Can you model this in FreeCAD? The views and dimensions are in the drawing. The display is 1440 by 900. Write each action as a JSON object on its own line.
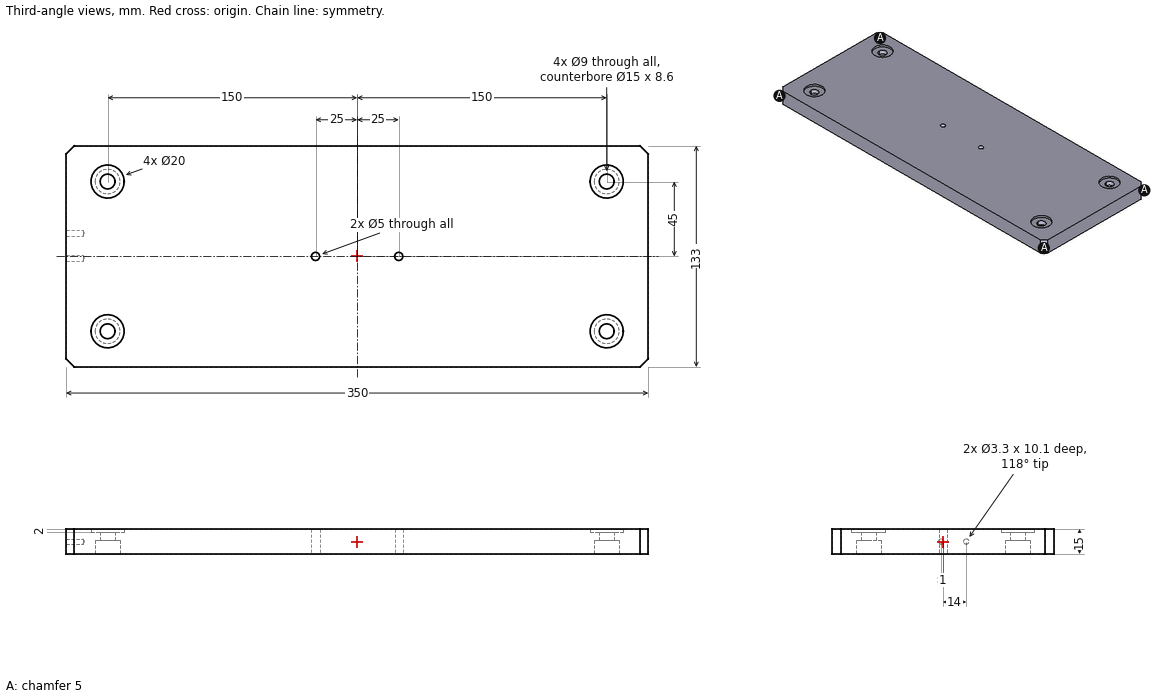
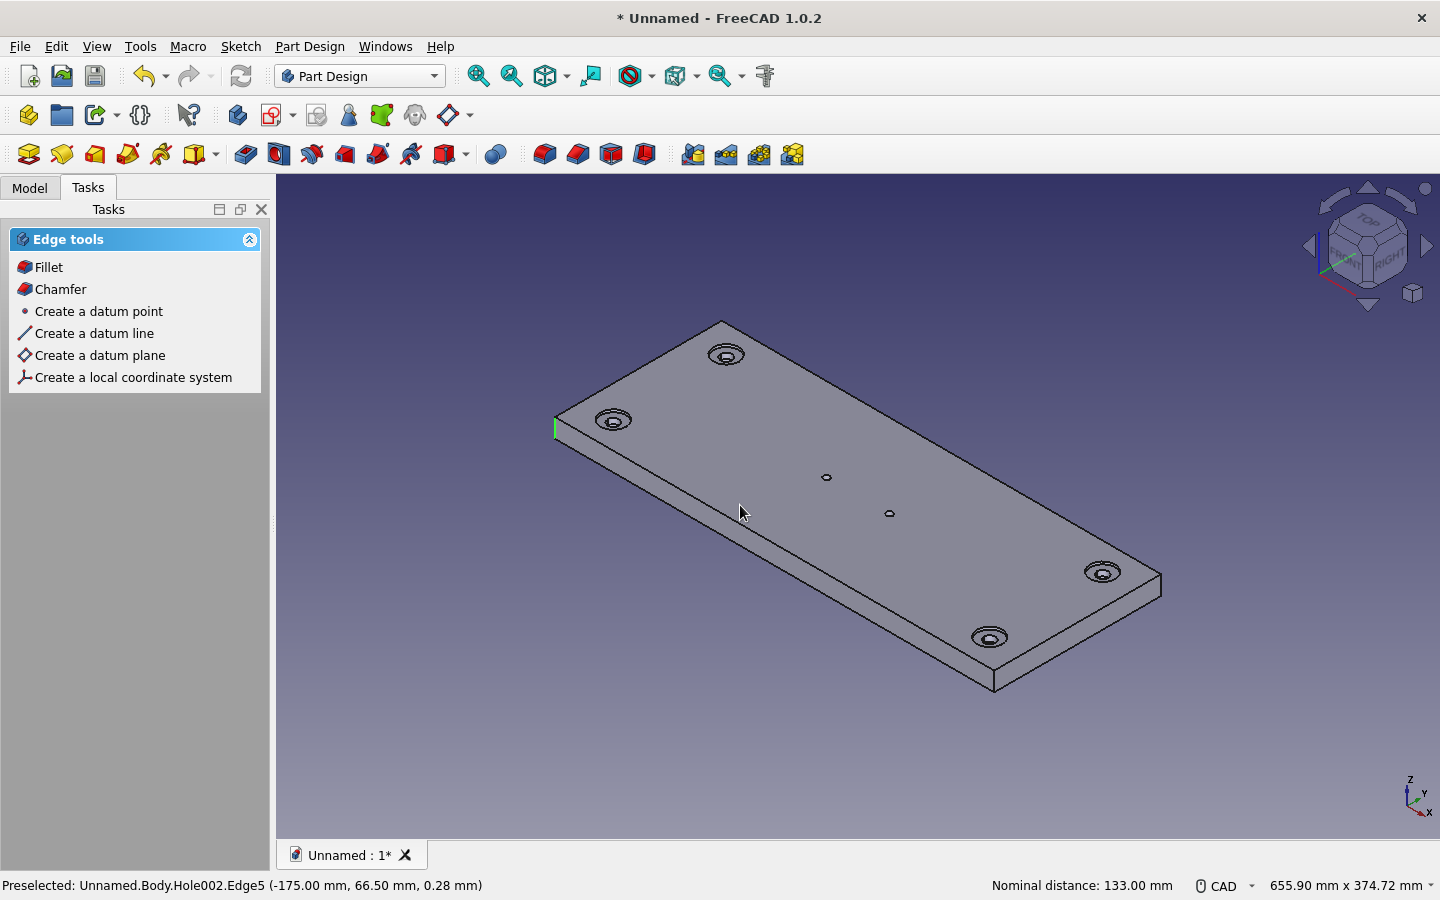
{"action": "left_click", "coordinate": [994, 680], "text": "ctrl"}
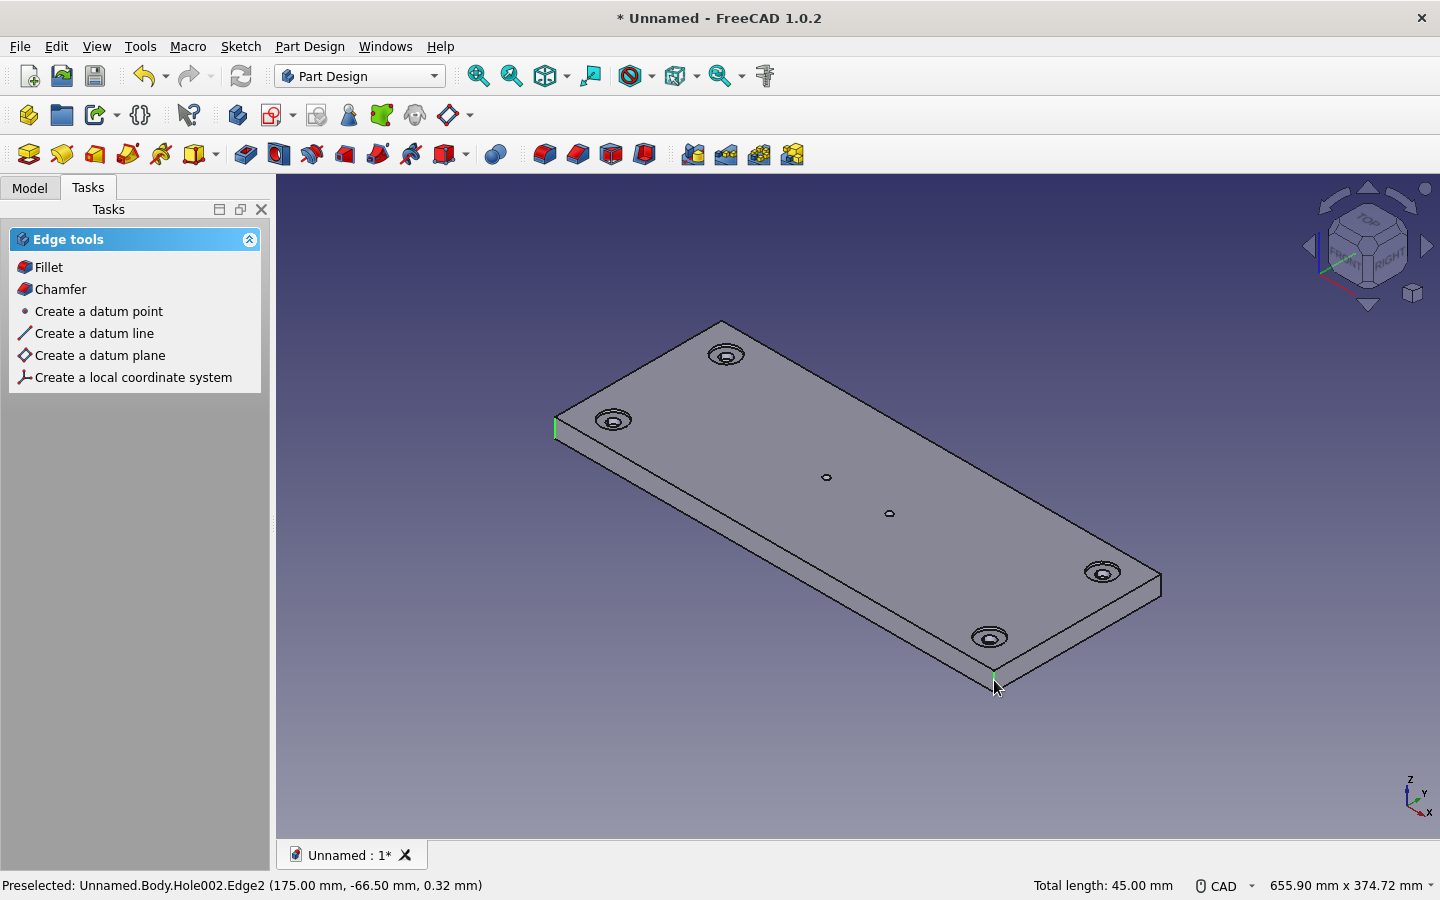
{"action": "key", "text": "2"}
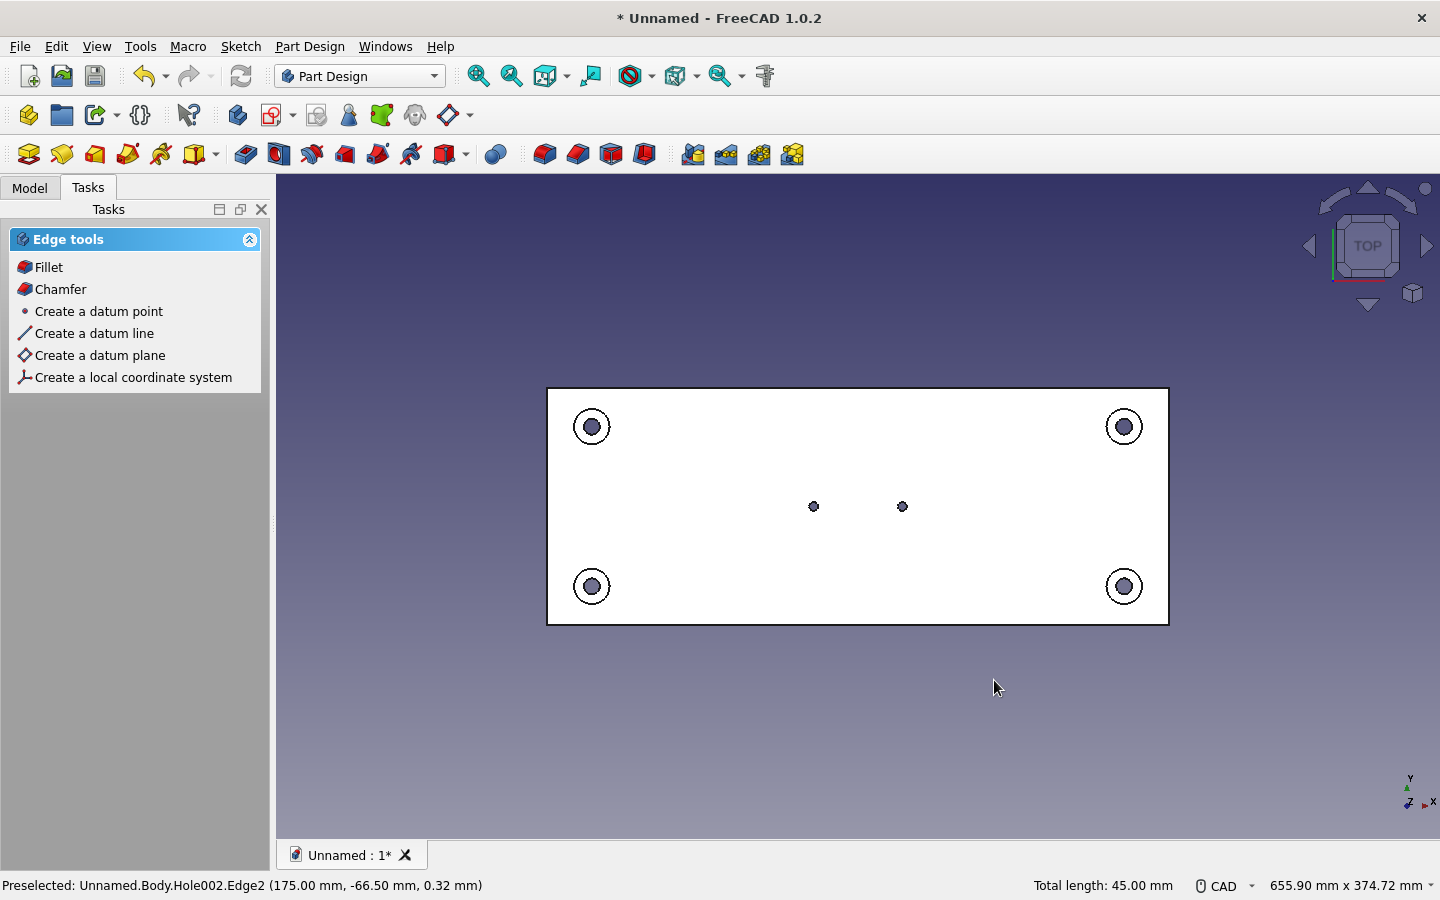
{"action": "key", "text": "1"}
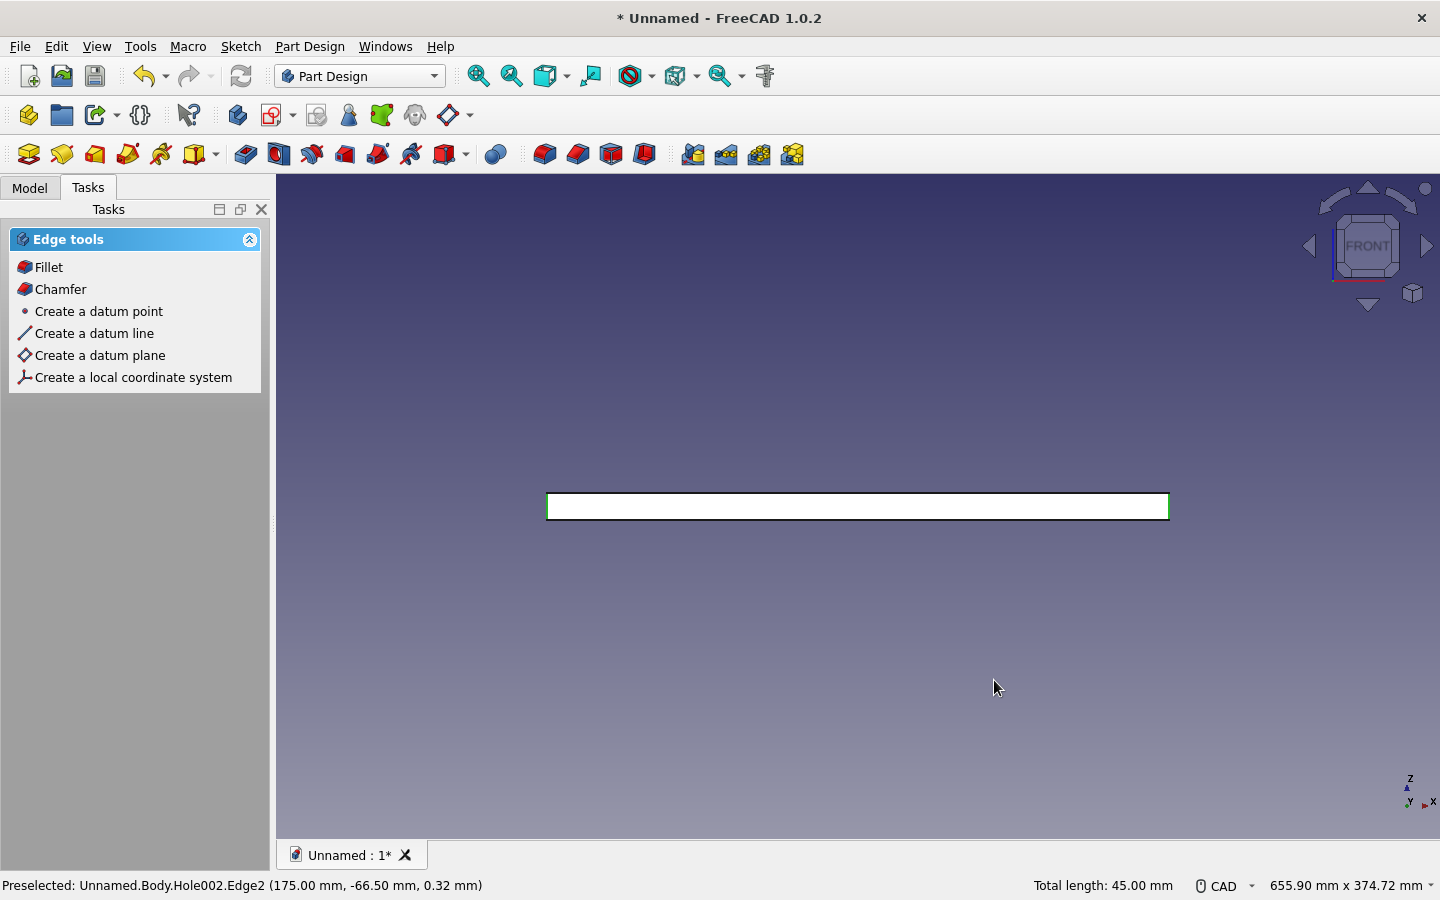
{"action": "key", "text": "3"}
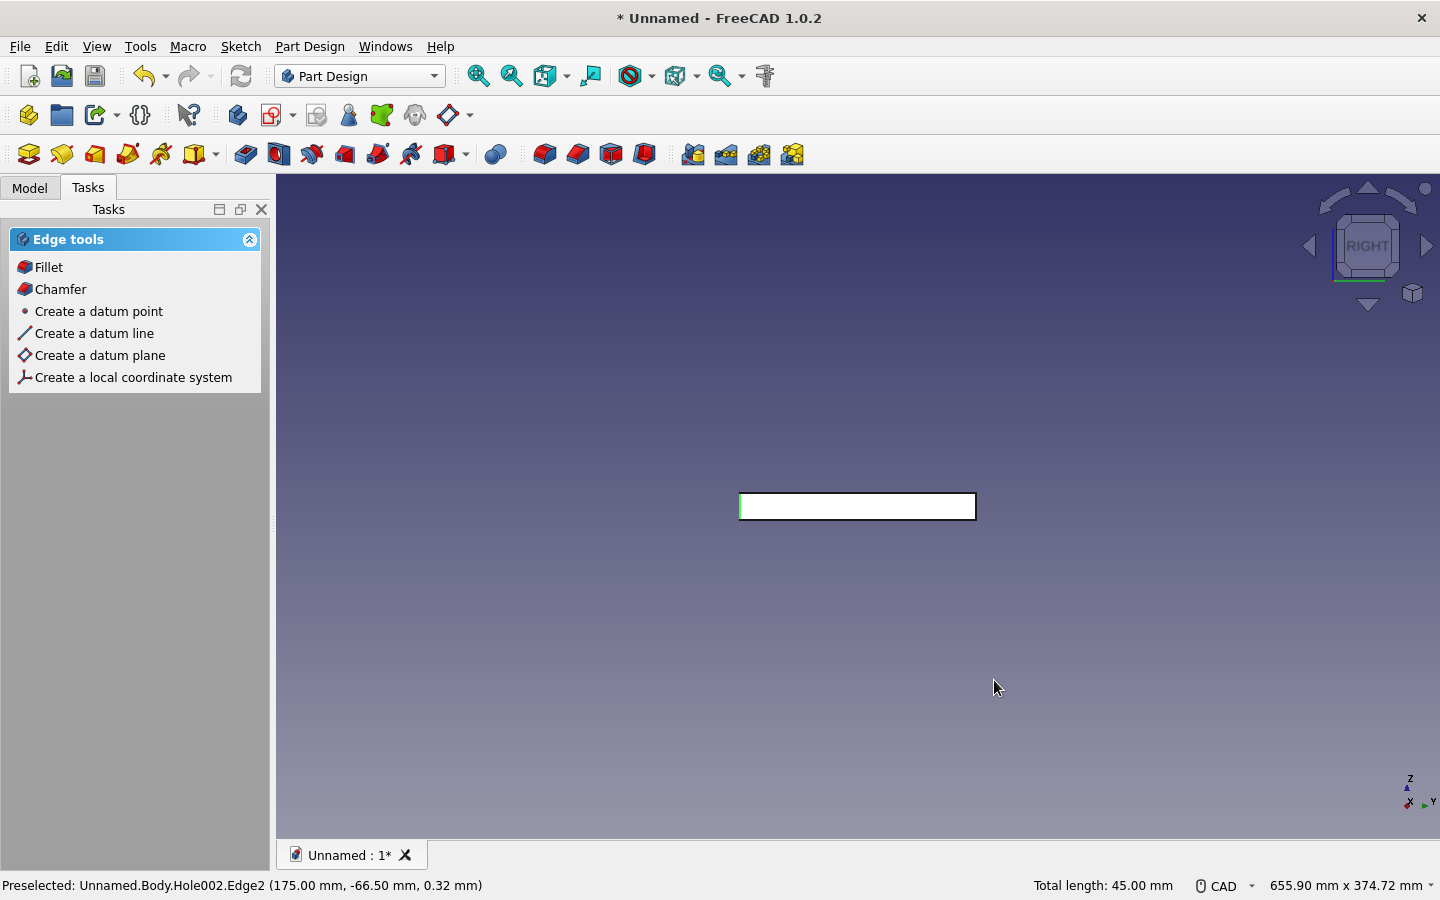
{"action": "key", "text": "v f"}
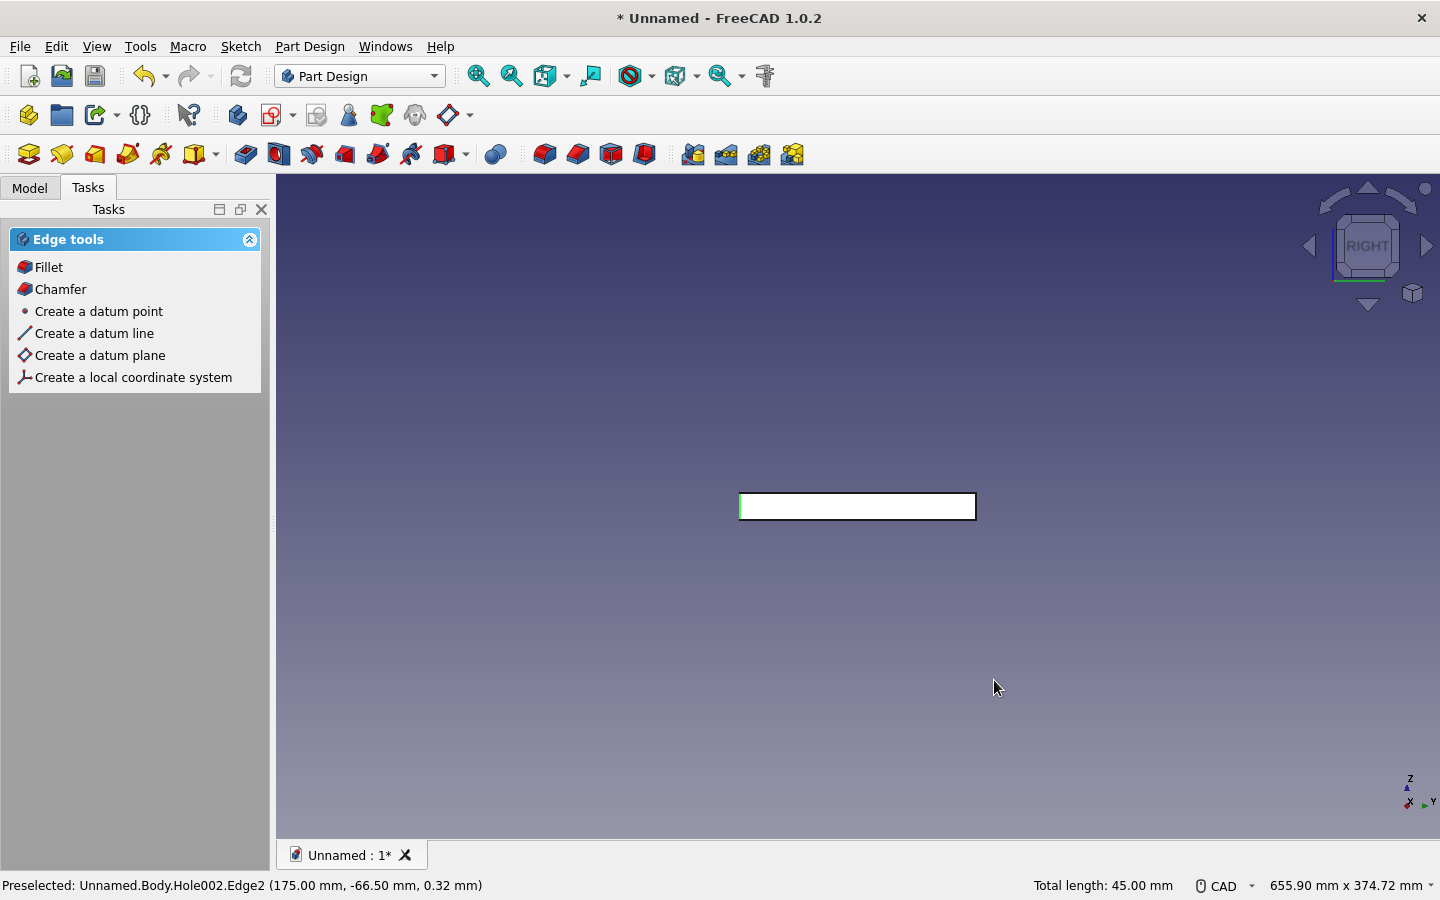
{"action": "left_click", "coordinate": [976, 505], "text": "ctrl"}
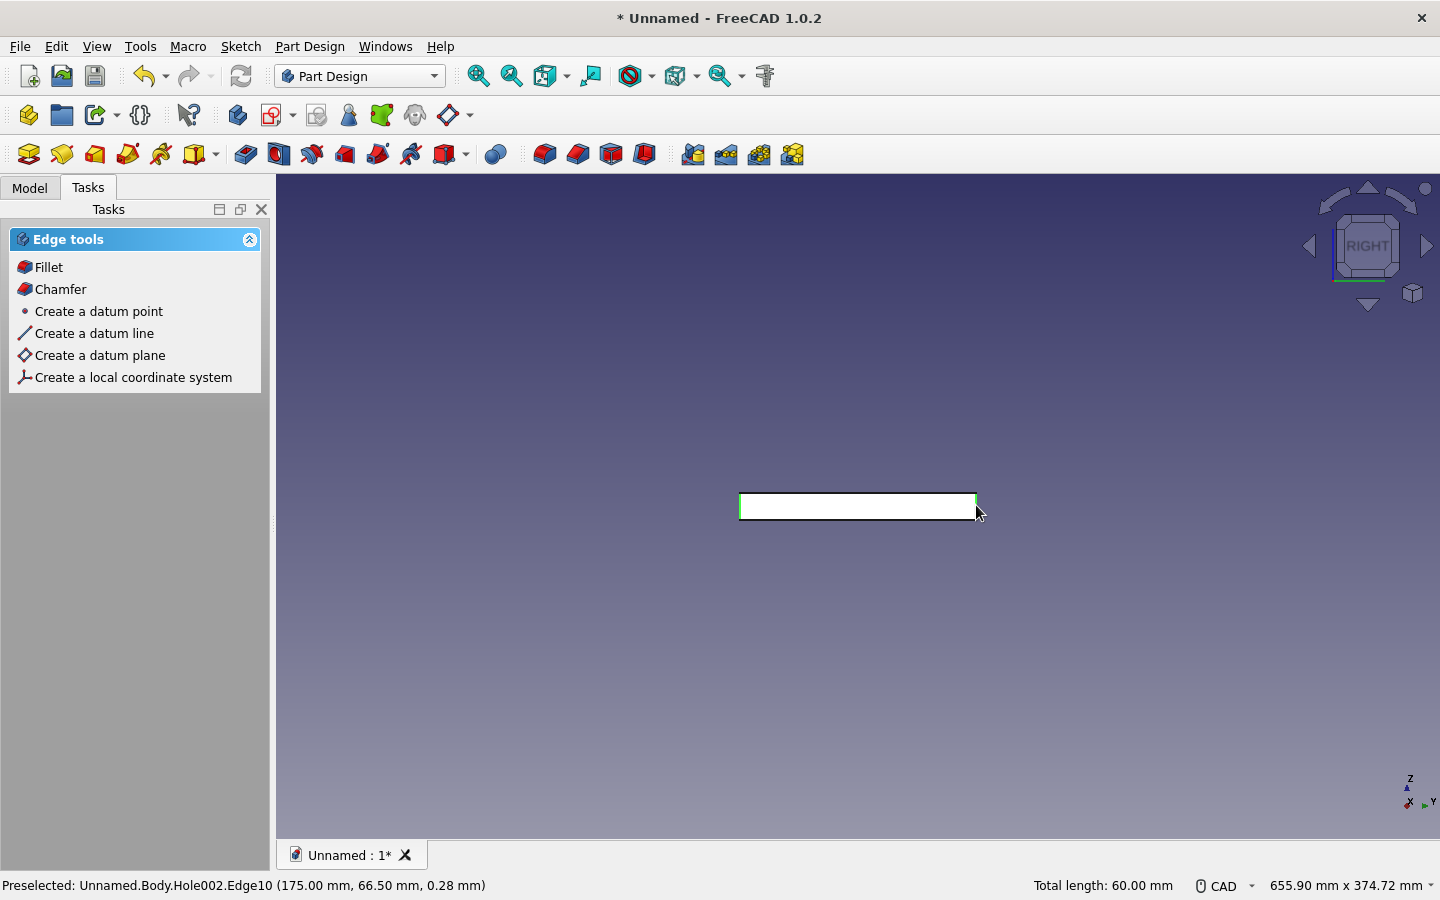
{"action": "left_click", "coordinate": [578, 154]}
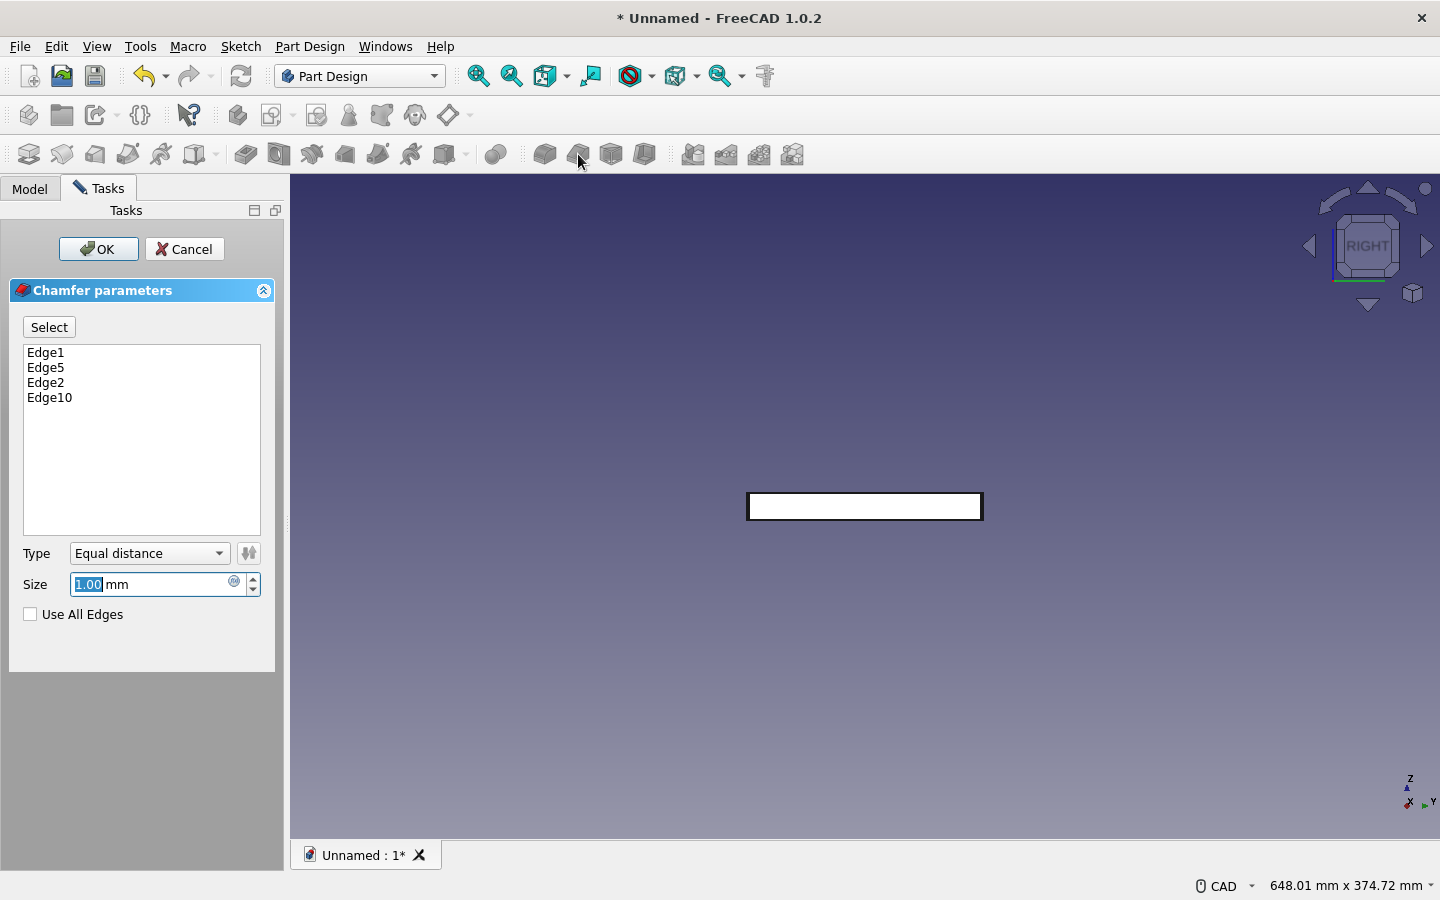
{"action": "type", "text": "5"}
{"action": "key", "text": "Tab"}